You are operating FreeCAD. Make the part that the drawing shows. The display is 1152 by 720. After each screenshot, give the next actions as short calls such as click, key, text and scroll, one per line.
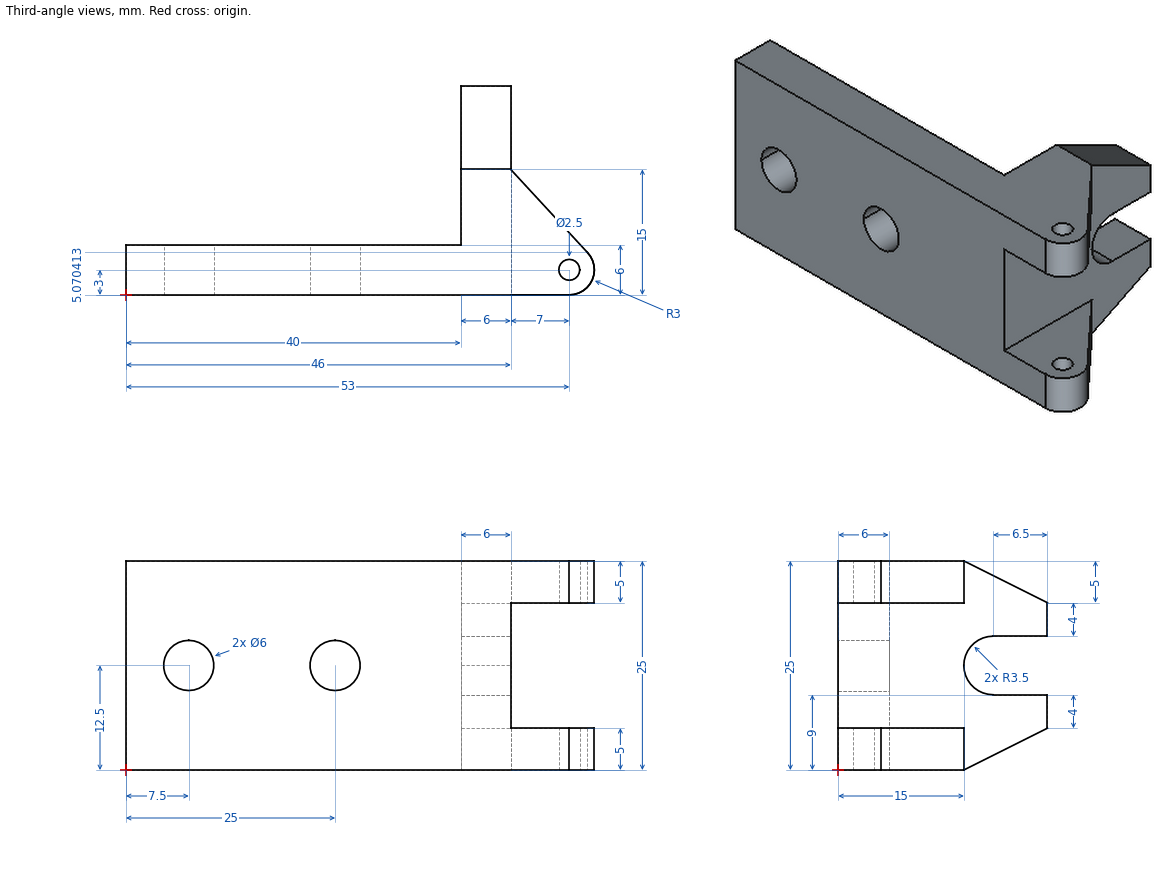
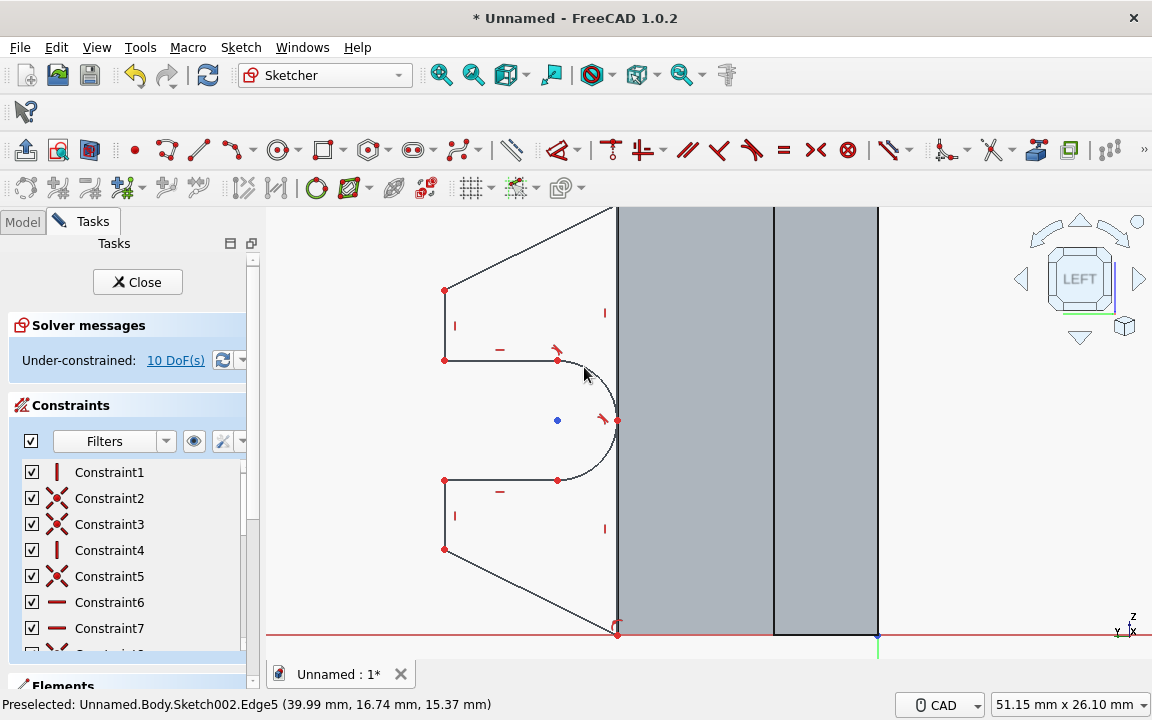
click(523, 480)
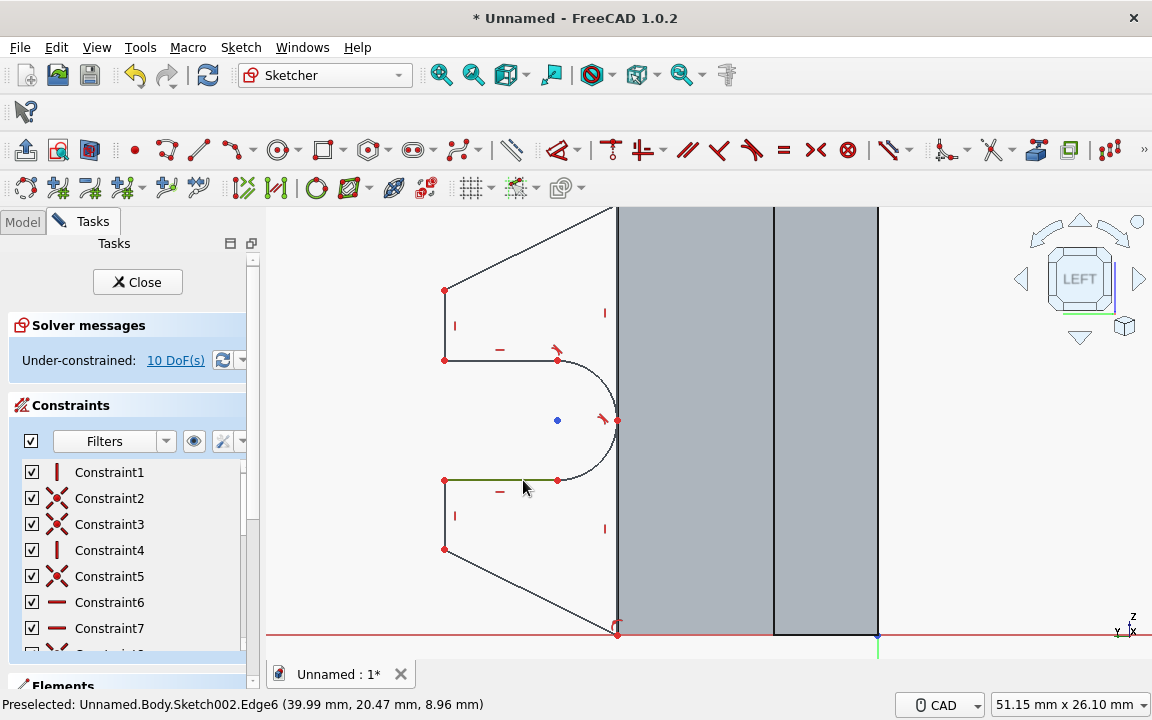
click(584, 474)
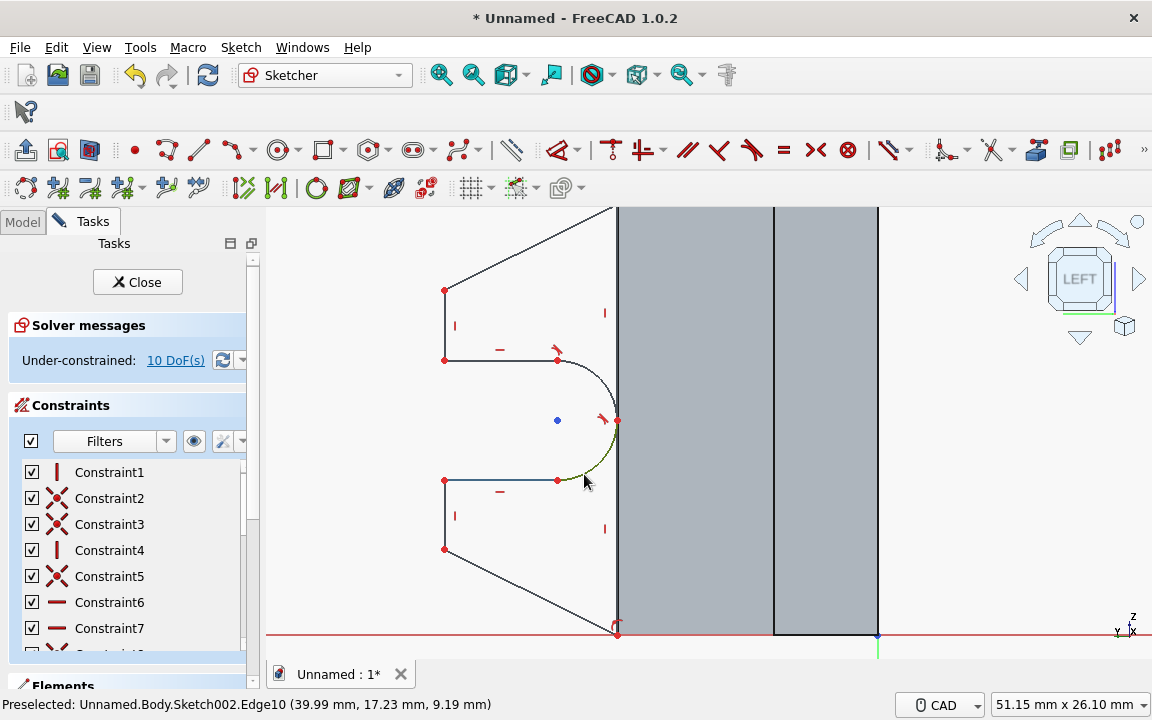
key(t)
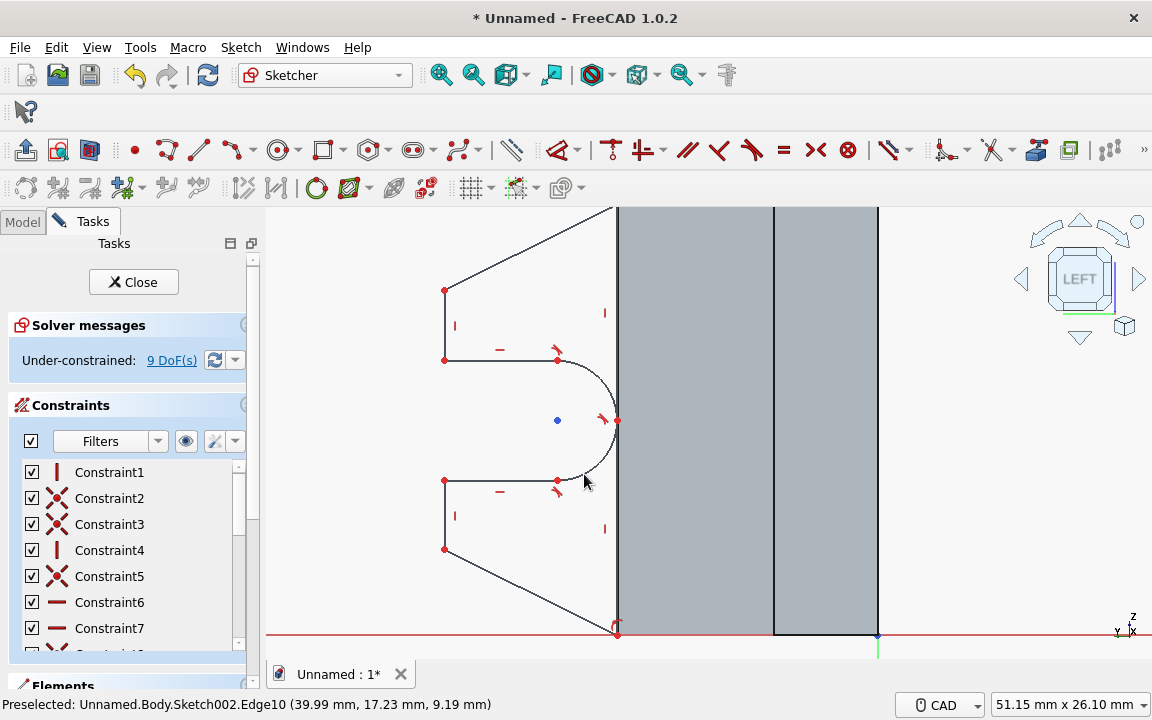
click(584, 367)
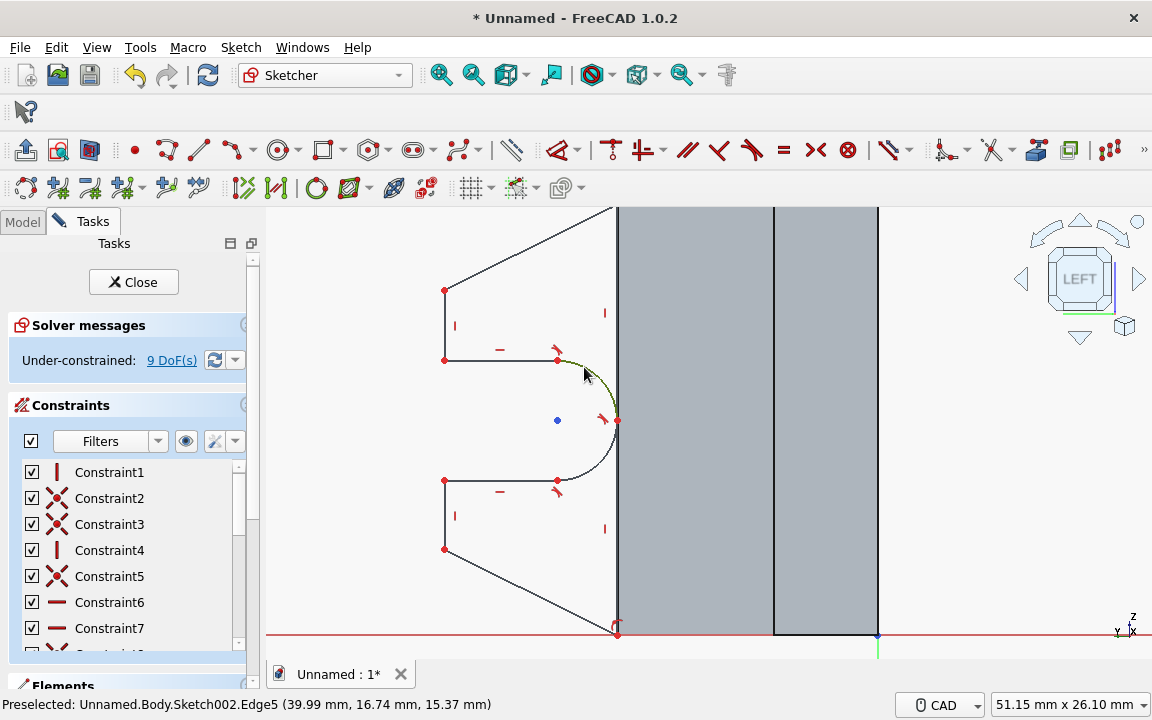
click(584, 474)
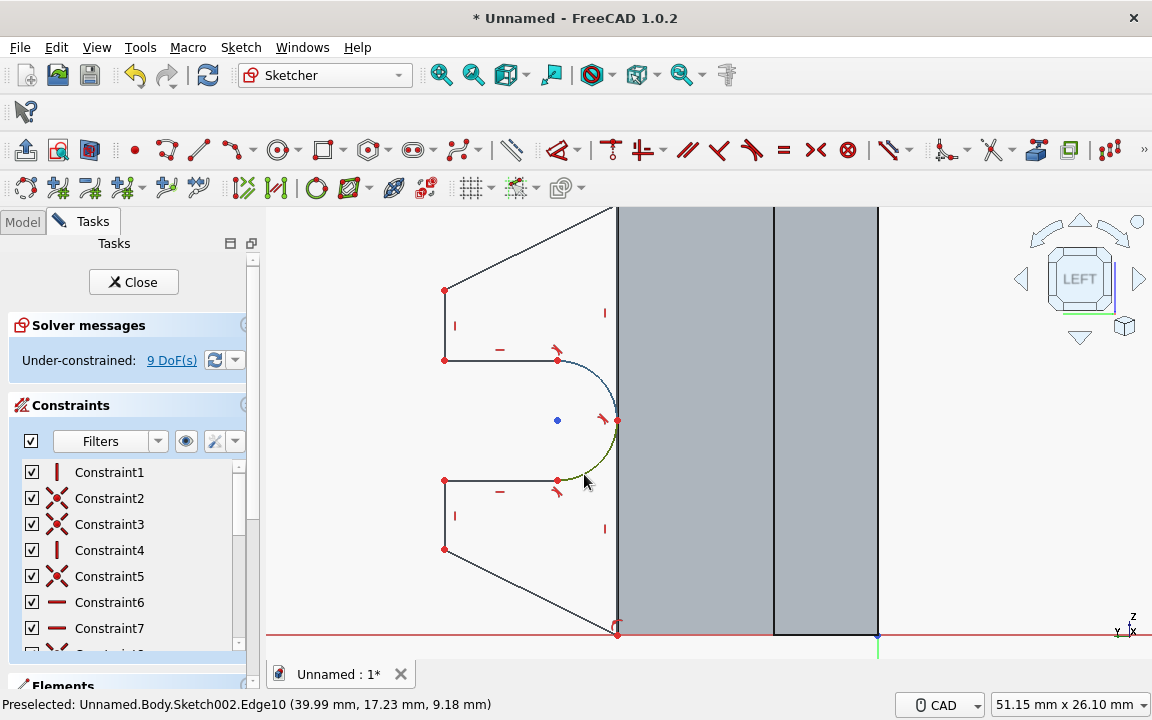
click(784, 150)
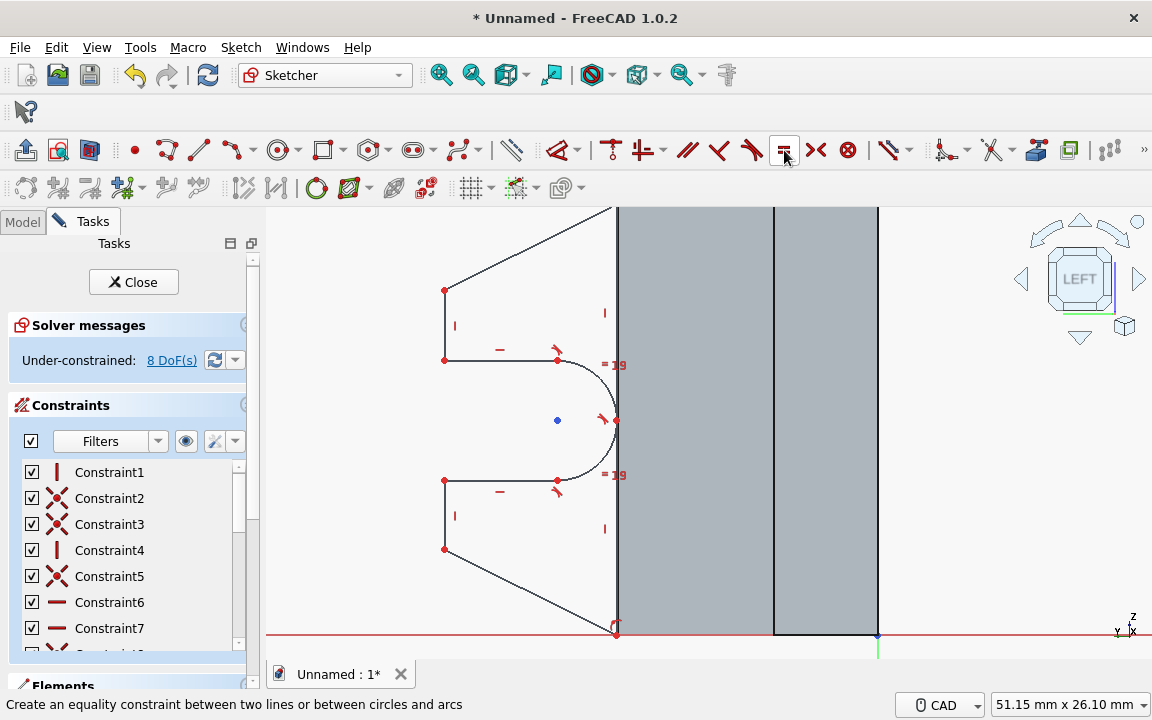
click(558, 150)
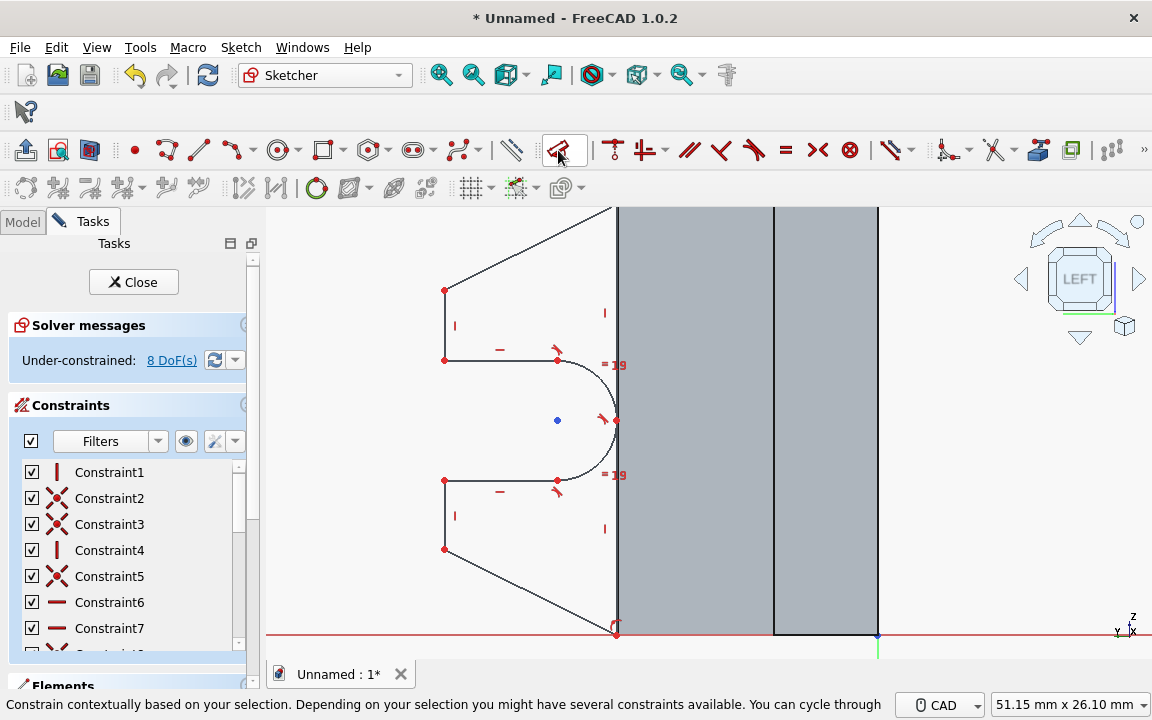
click(584, 367)
click(598, 338)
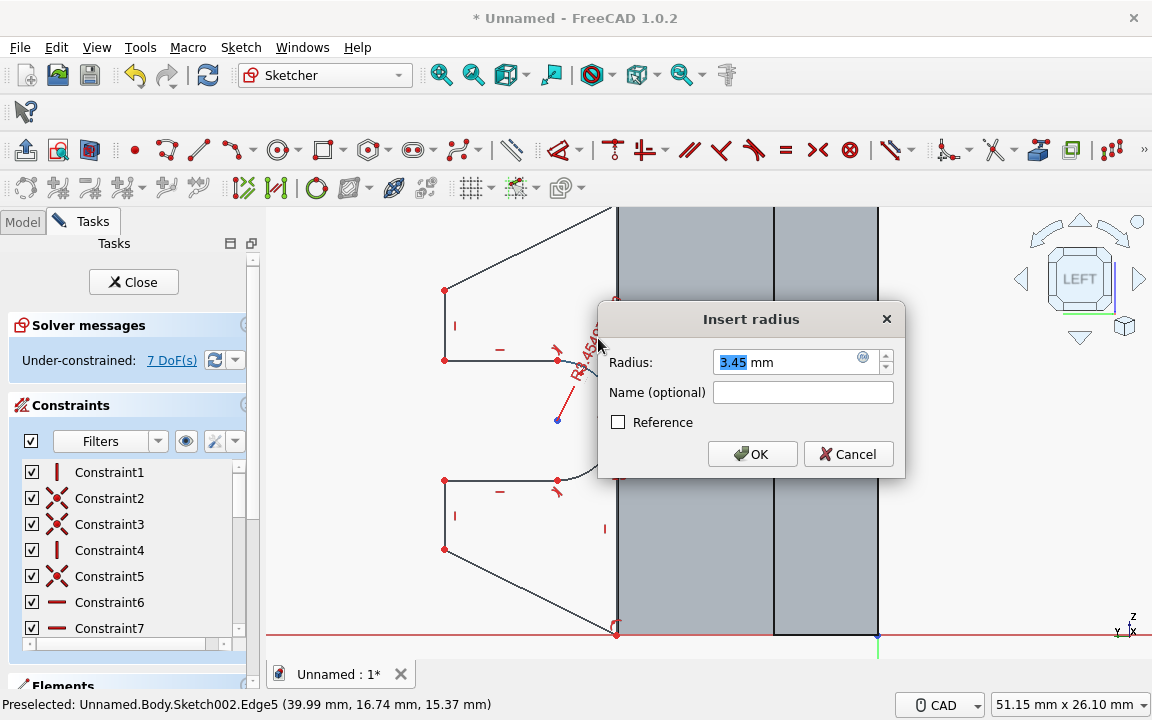
text(3.5)
key(Return)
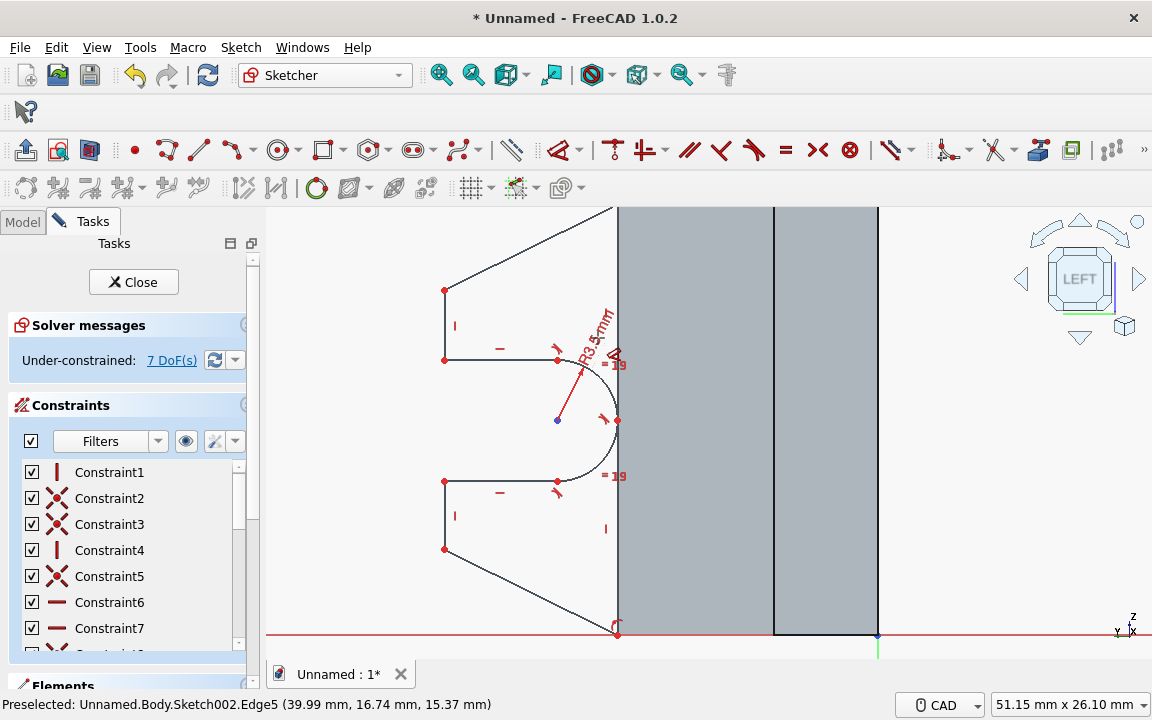
click(445, 311)
click(411, 325)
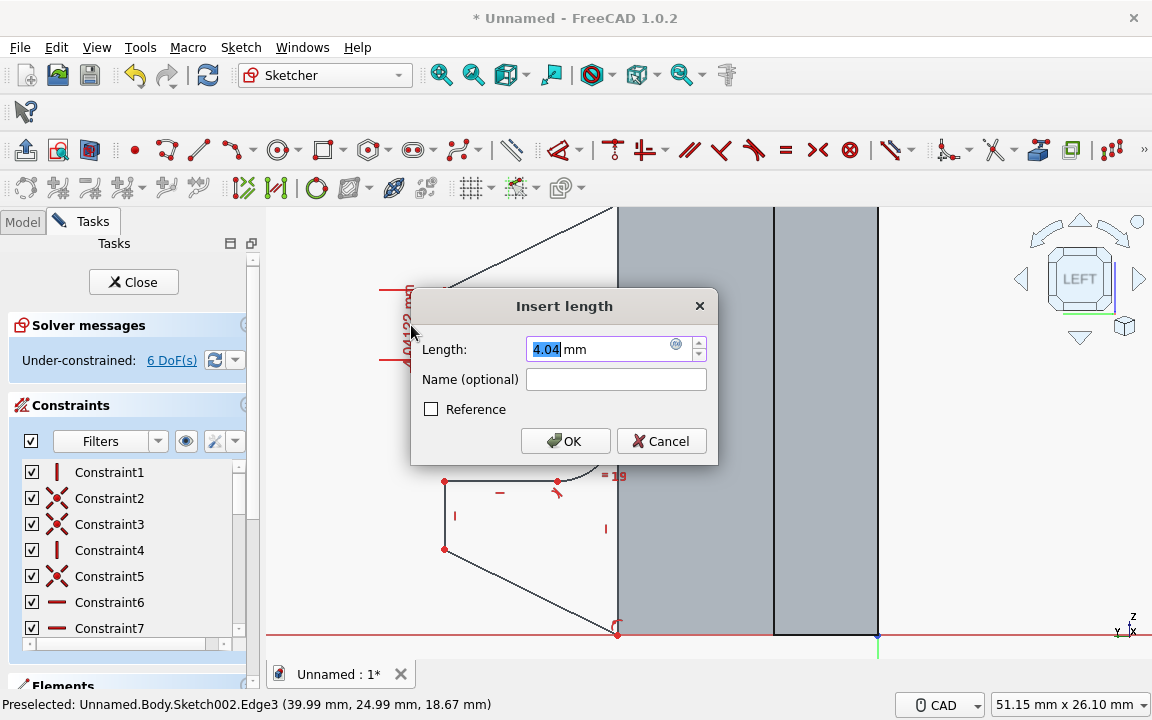
text(4)
key(Return)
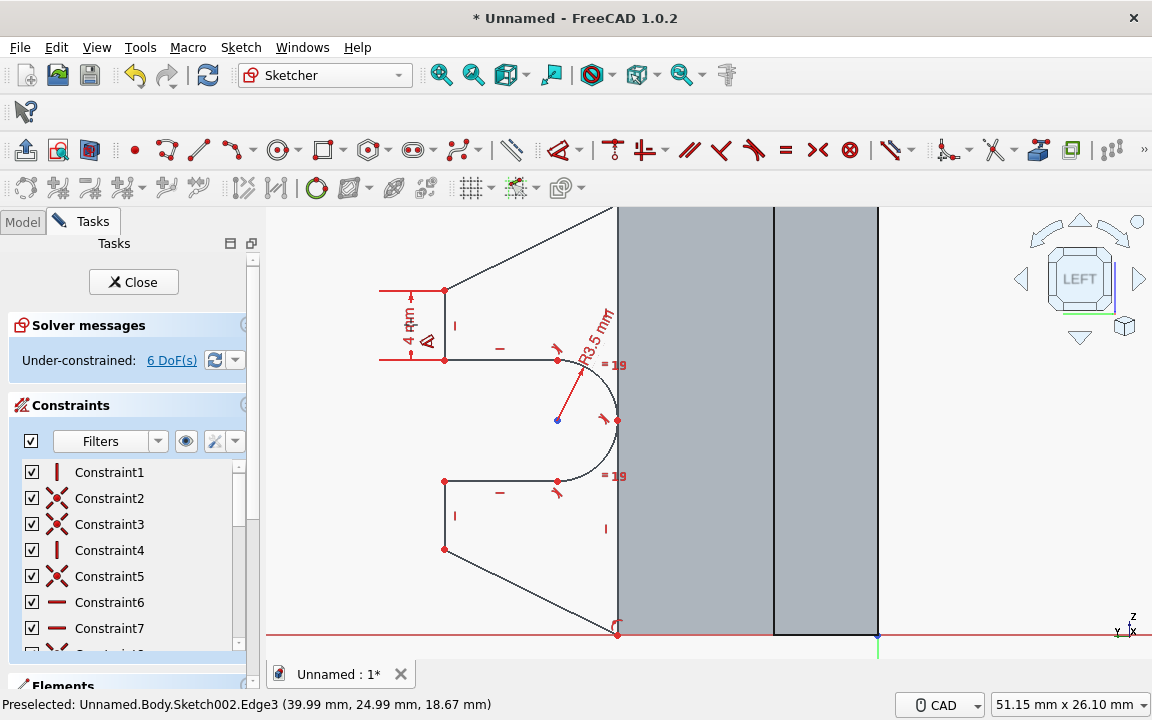
click(445, 502)
click(411, 516)